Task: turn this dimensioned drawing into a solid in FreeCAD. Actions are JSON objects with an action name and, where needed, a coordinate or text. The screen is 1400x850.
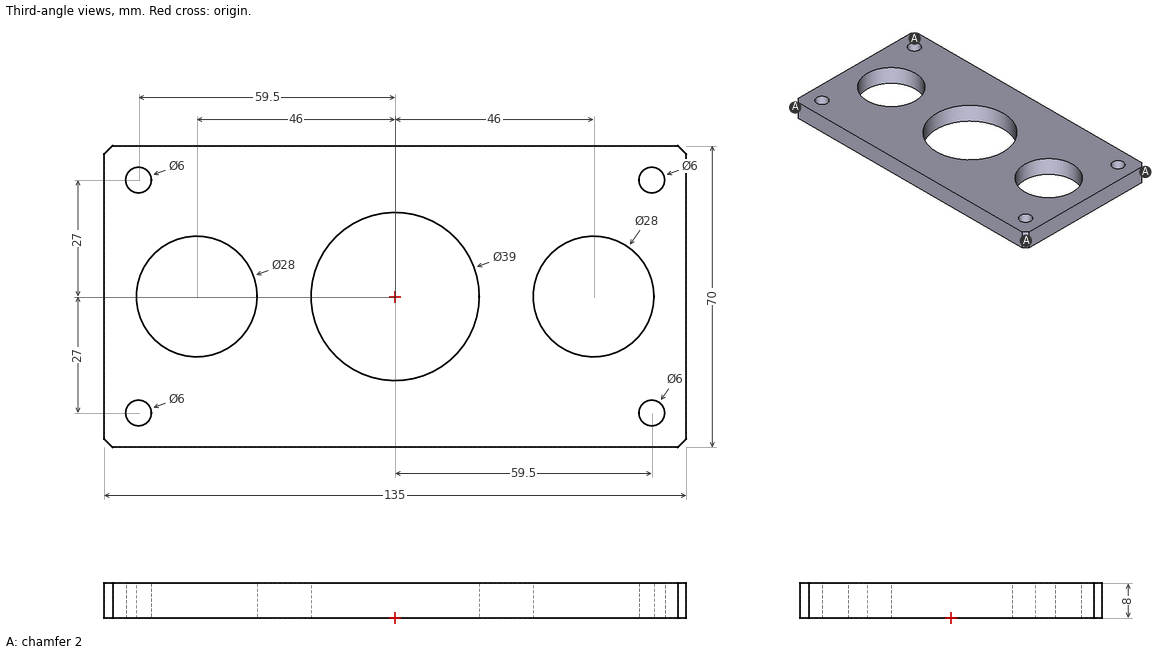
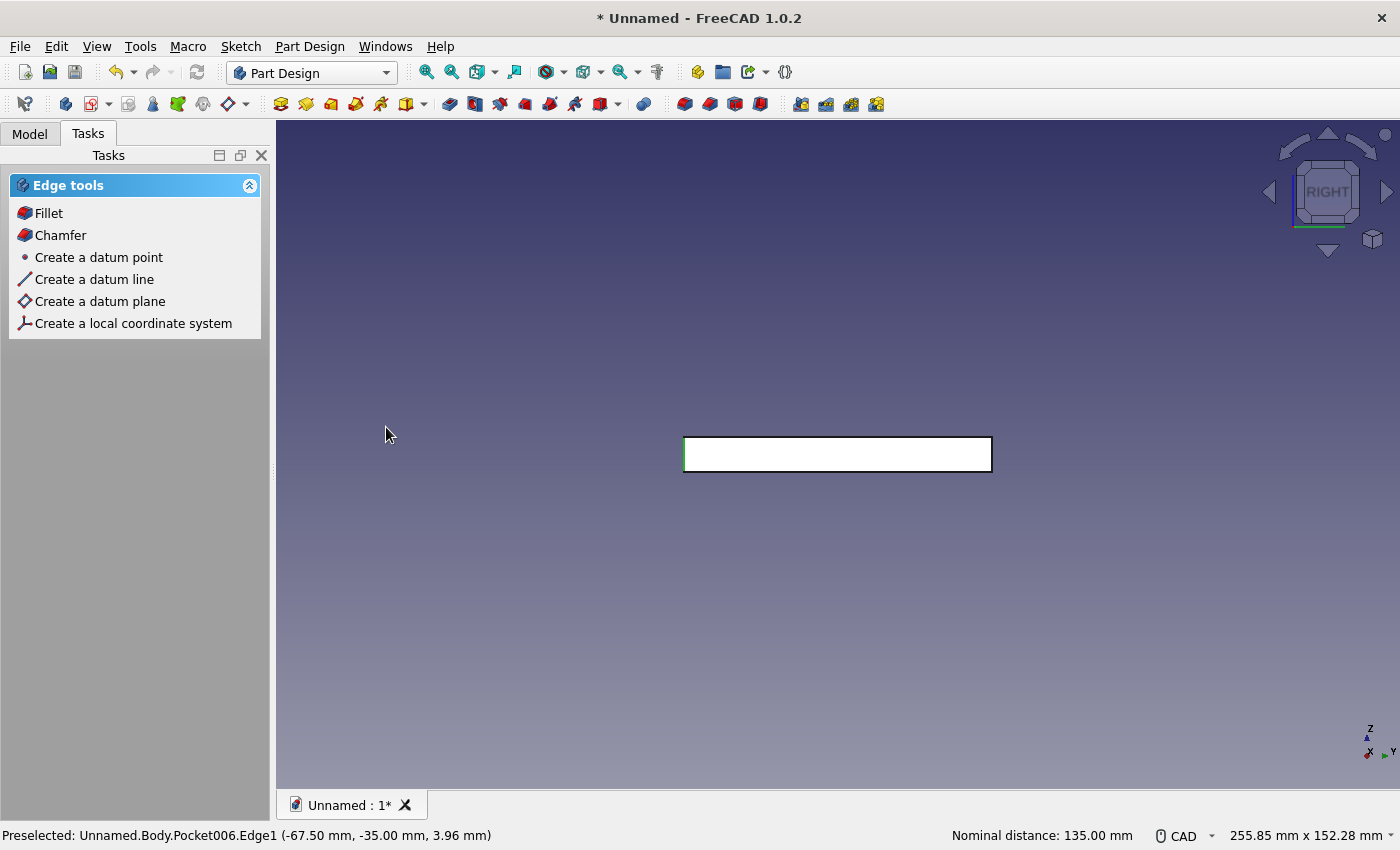
{"action": "left_click", "coordinate": [992, 453], "text": "ctrl"}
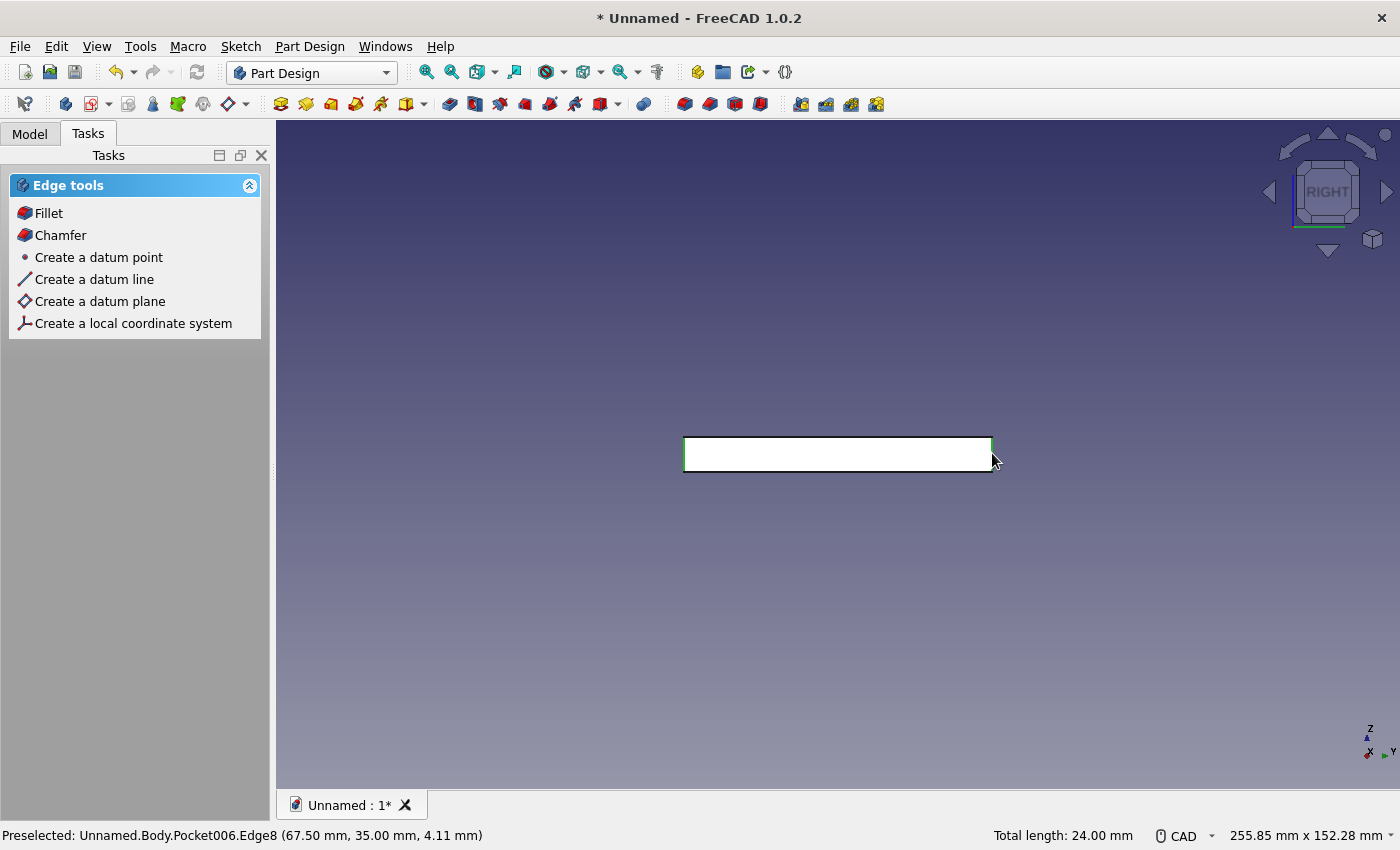
{"action": "key", "text": "5"}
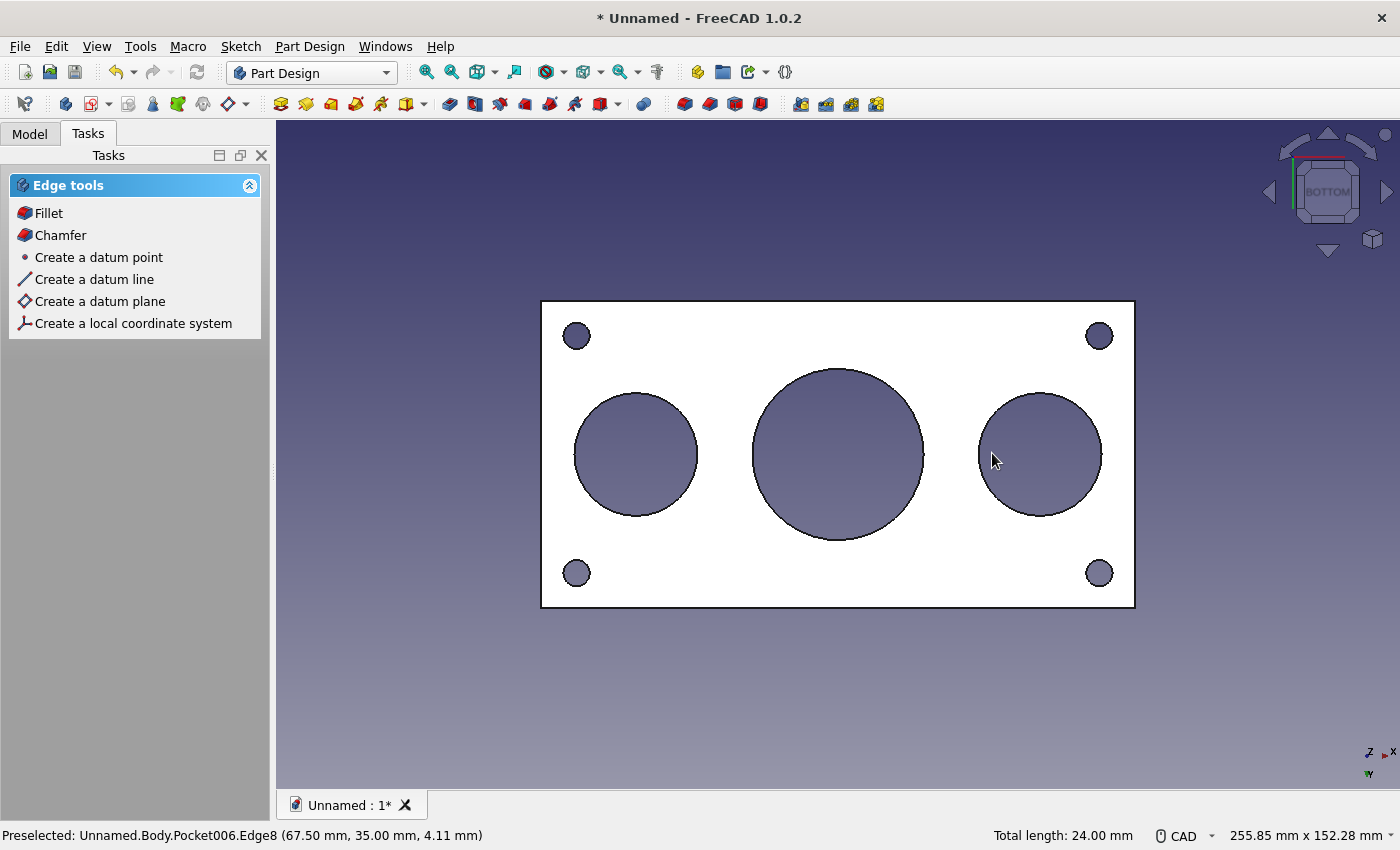
{"action": "key", "text": "4"}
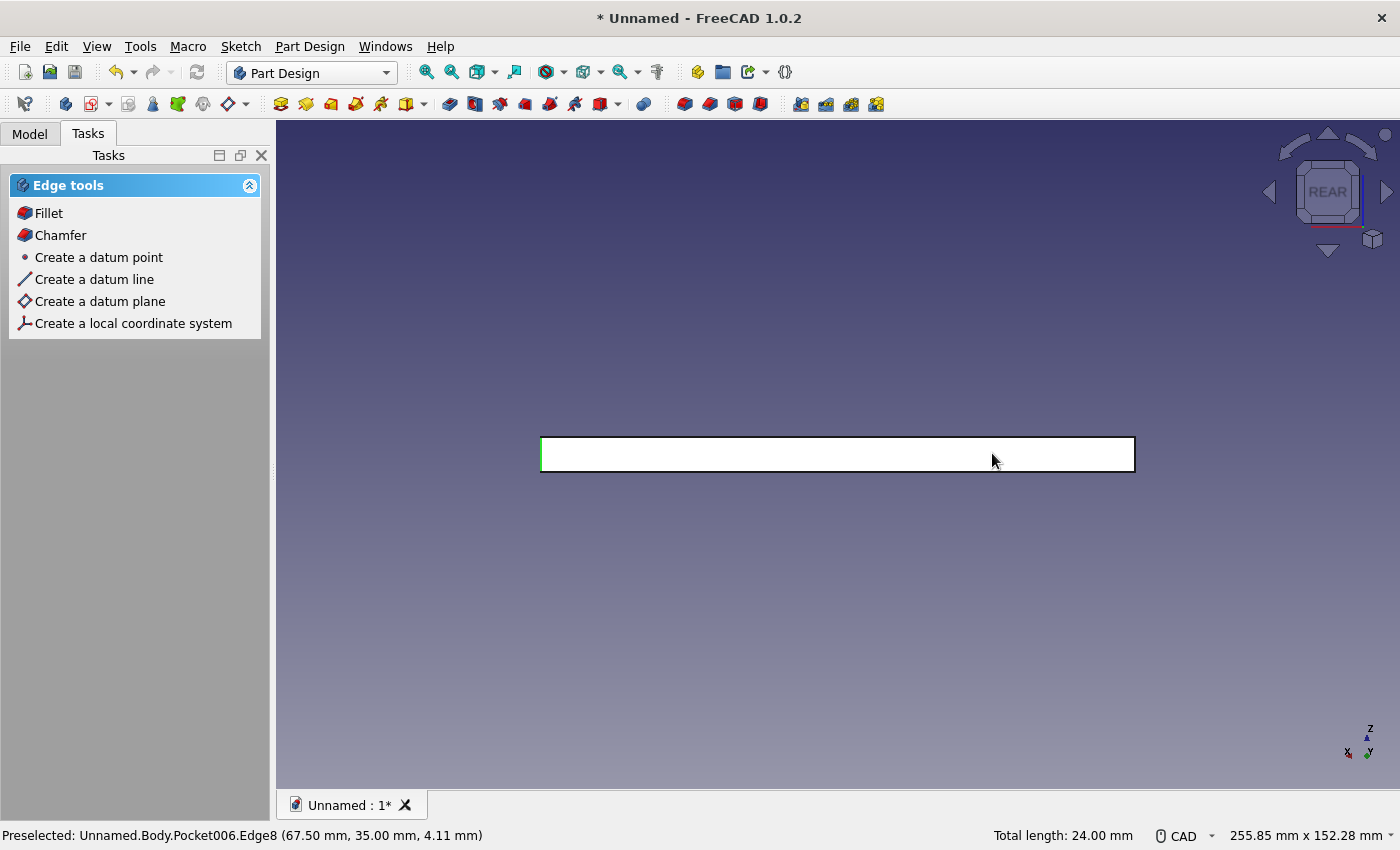
{"action": "left_click", "coordinate": [1135, 453], "text": "ctrl"}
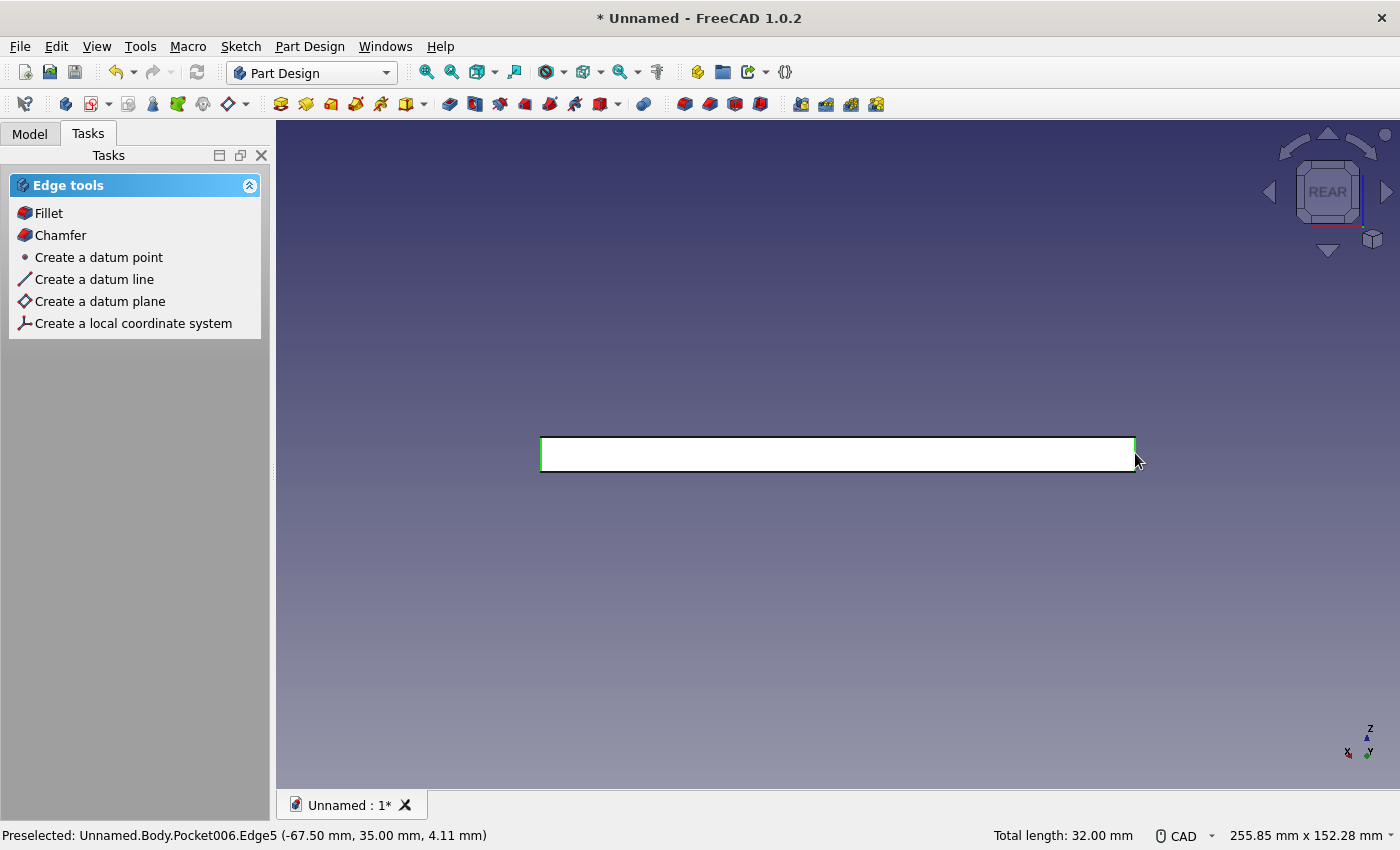
{"action": "left_click", "coordinate": [710, 104]}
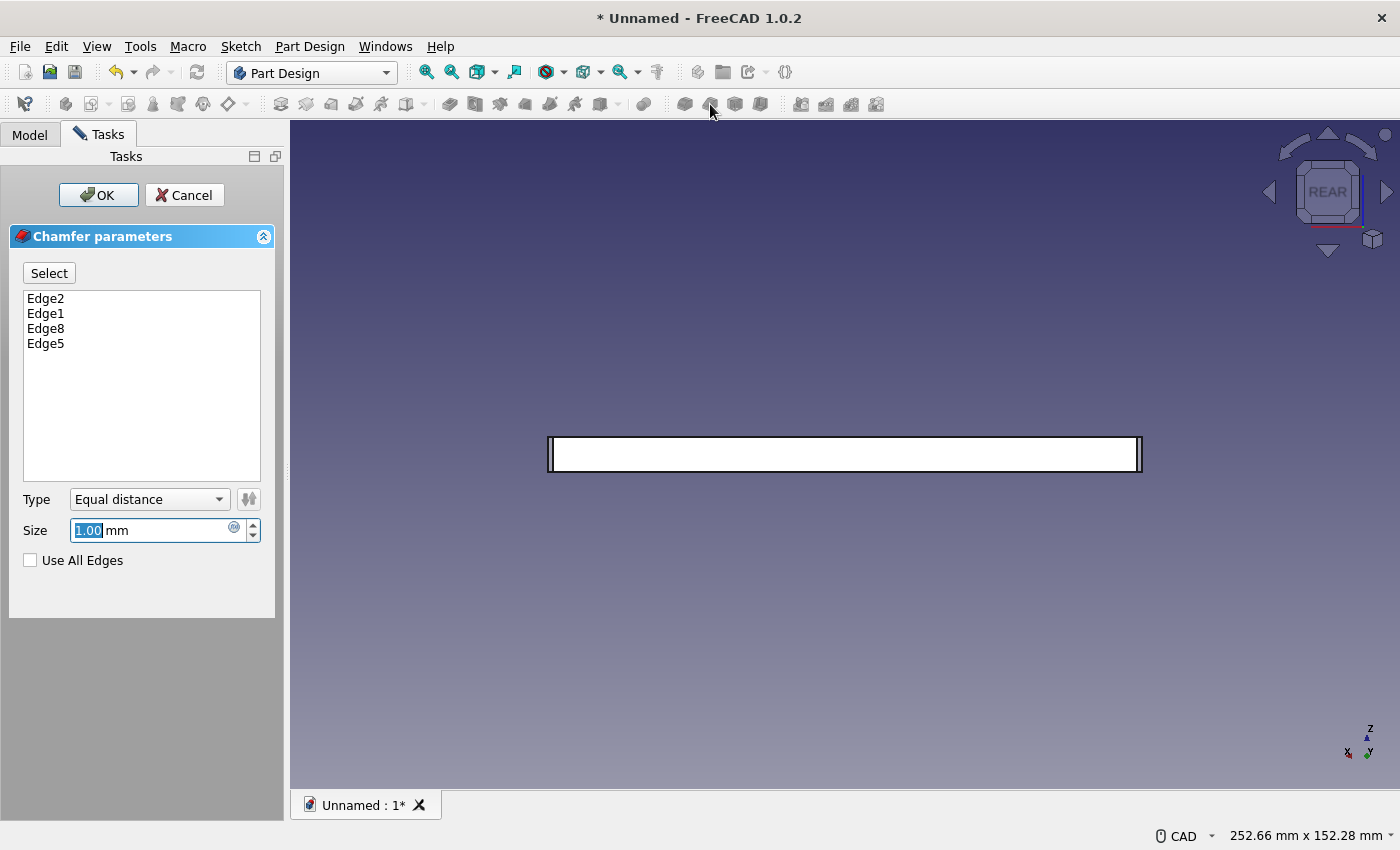
{"action": "type", "text": "2"}
{"action": "key", "text": "Tab"}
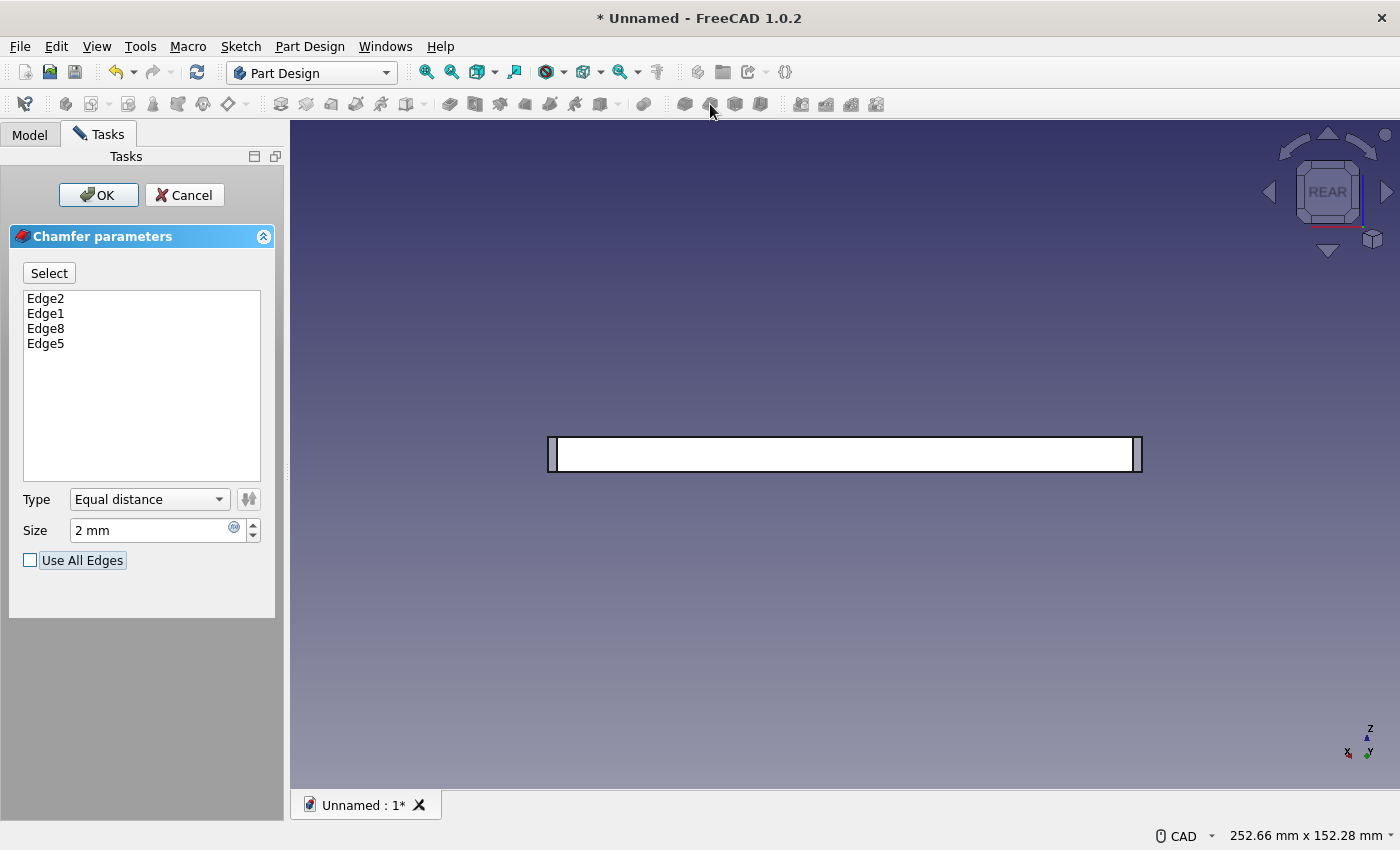
{"action": "left_click", "coordinate": [99, 195]}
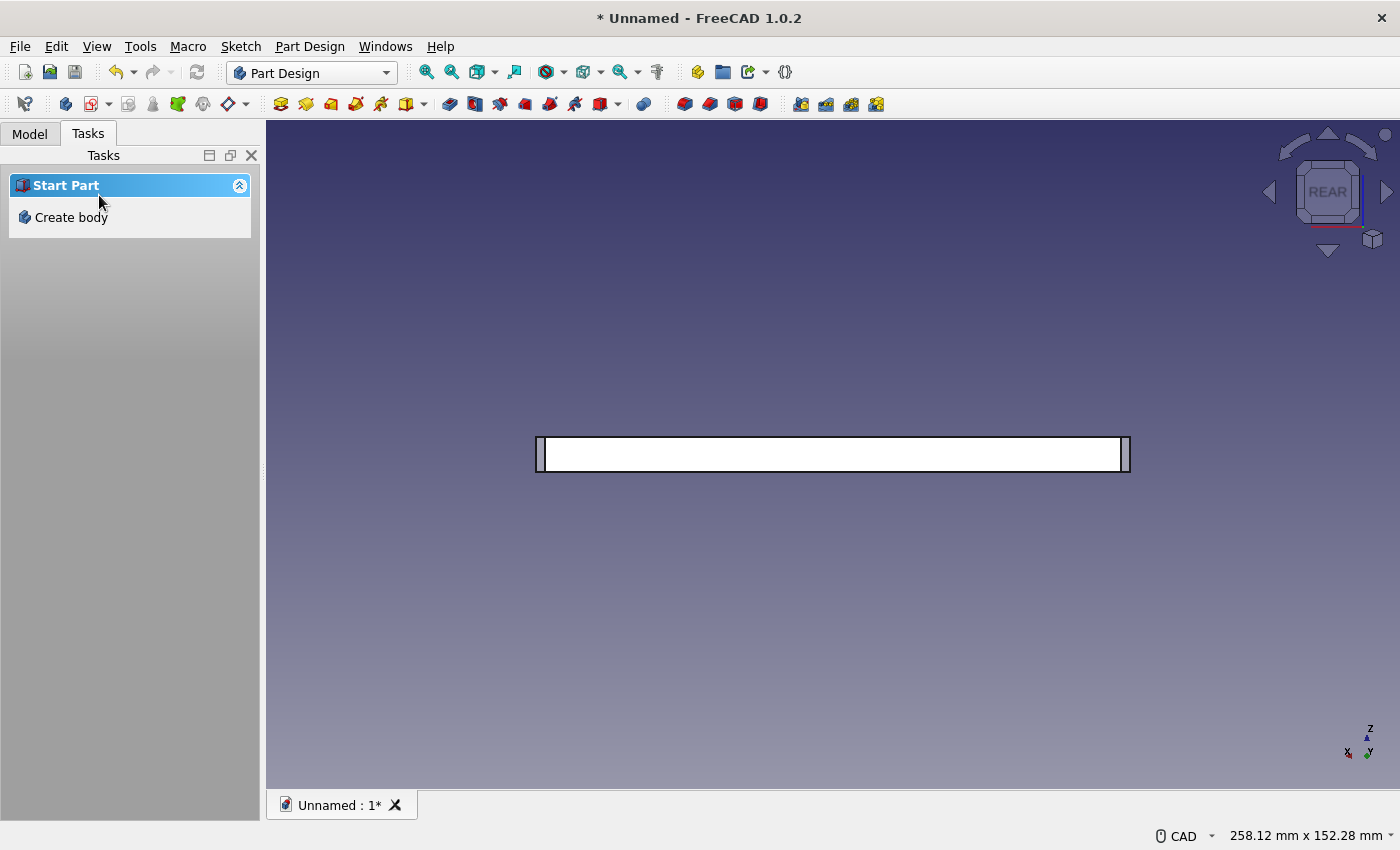
{"action": "key", "text": "0"}